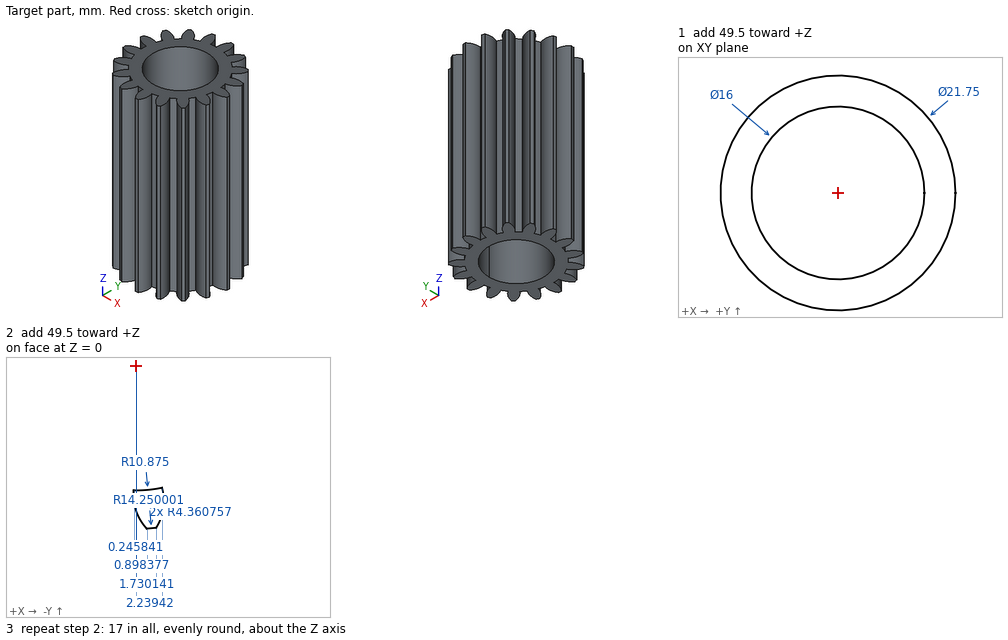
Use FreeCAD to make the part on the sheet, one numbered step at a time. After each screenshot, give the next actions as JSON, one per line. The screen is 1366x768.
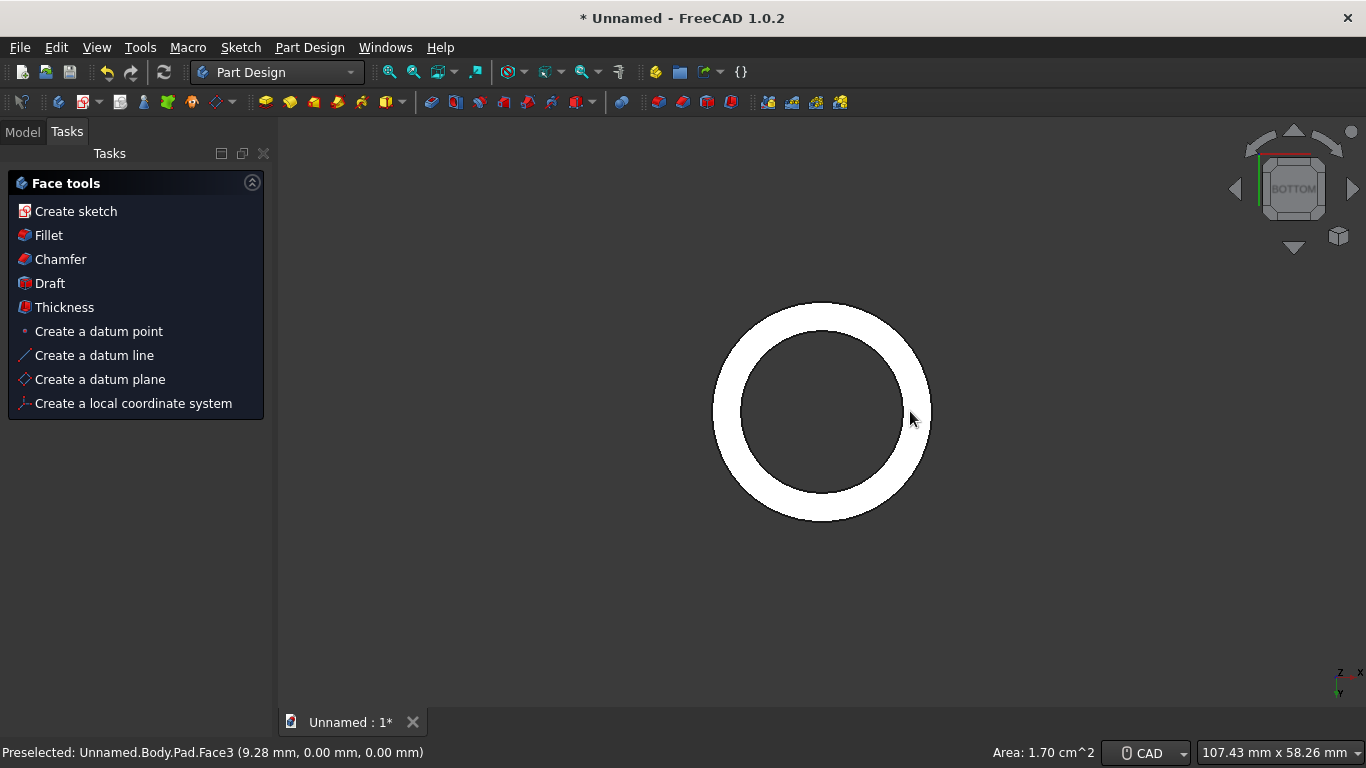
{"action": "left_click", "coordinate": [84, 102]}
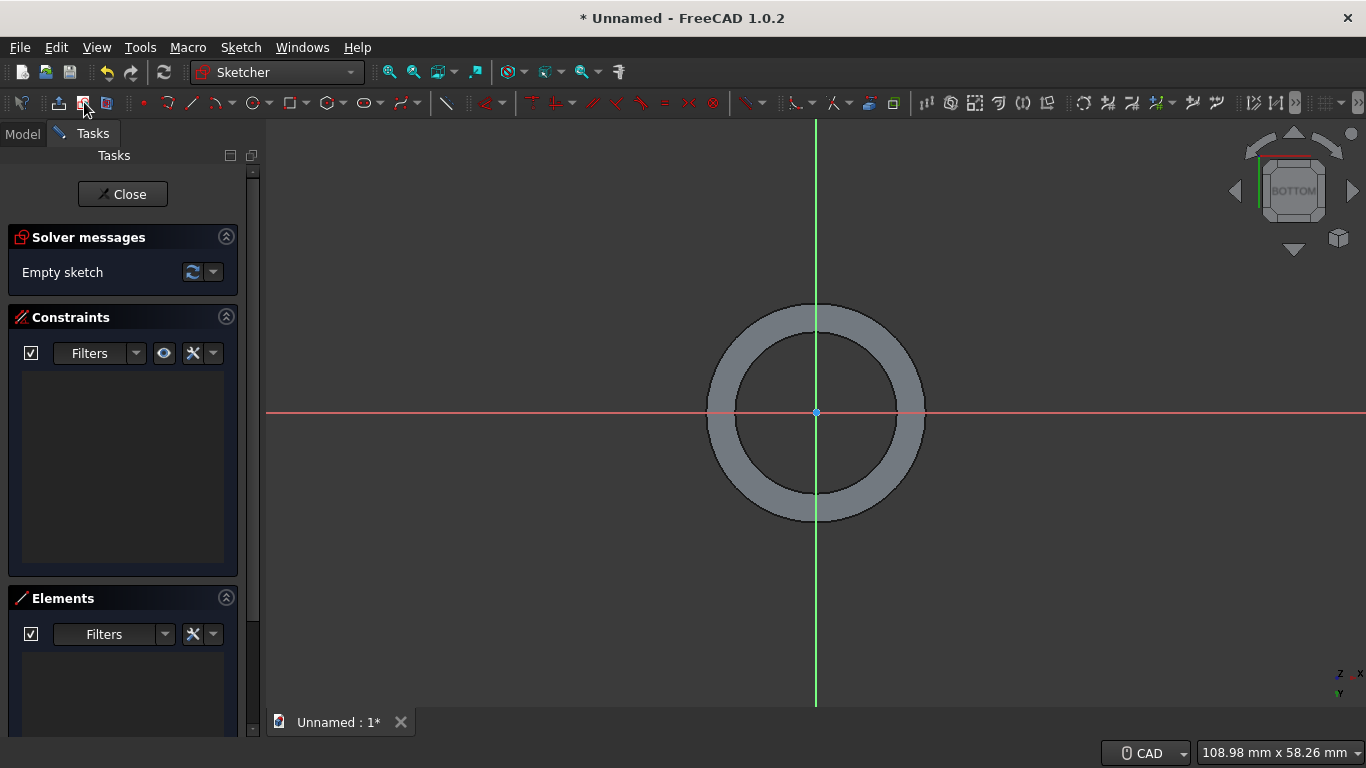
{"action": "scroll", "coordinate": [835, 551], "scroll_direction": "up", "scroll_amount": 12}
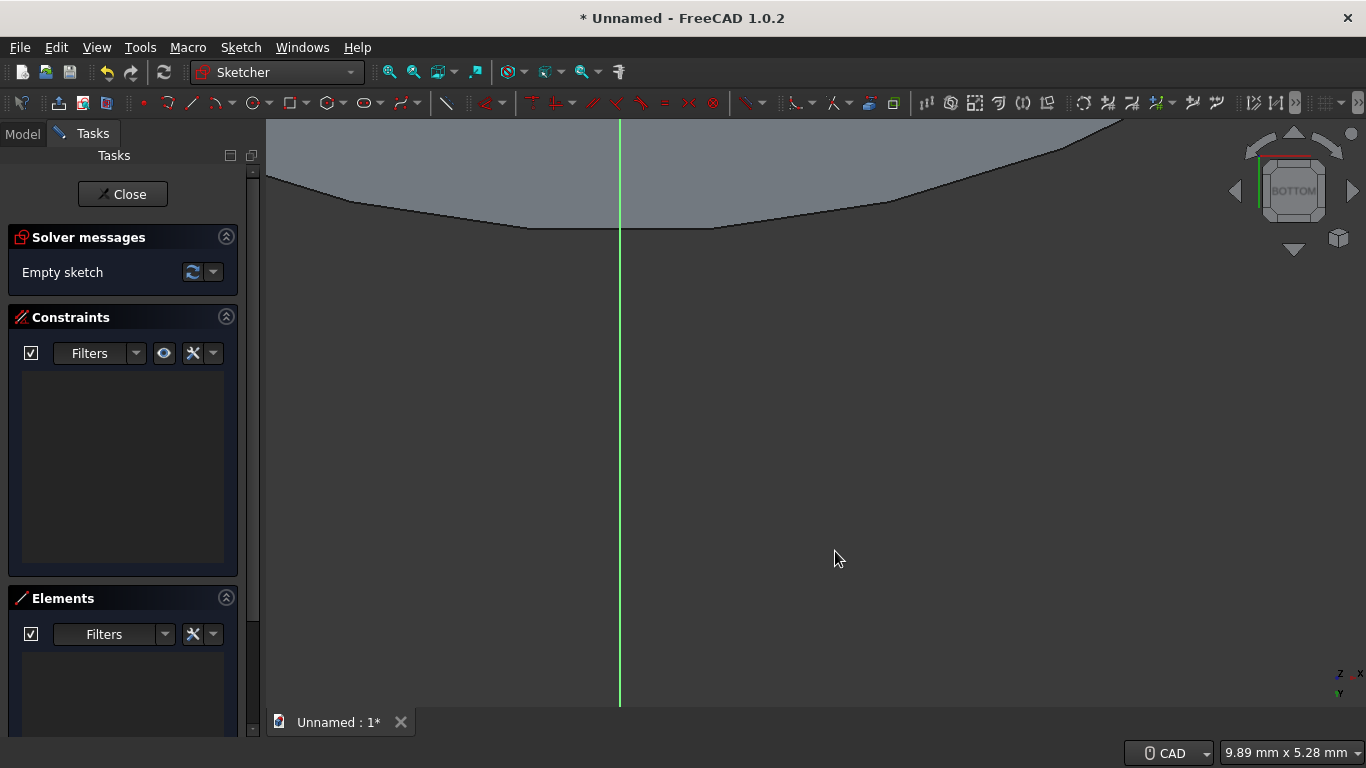
{"action": "key", "text": "g 3 a"}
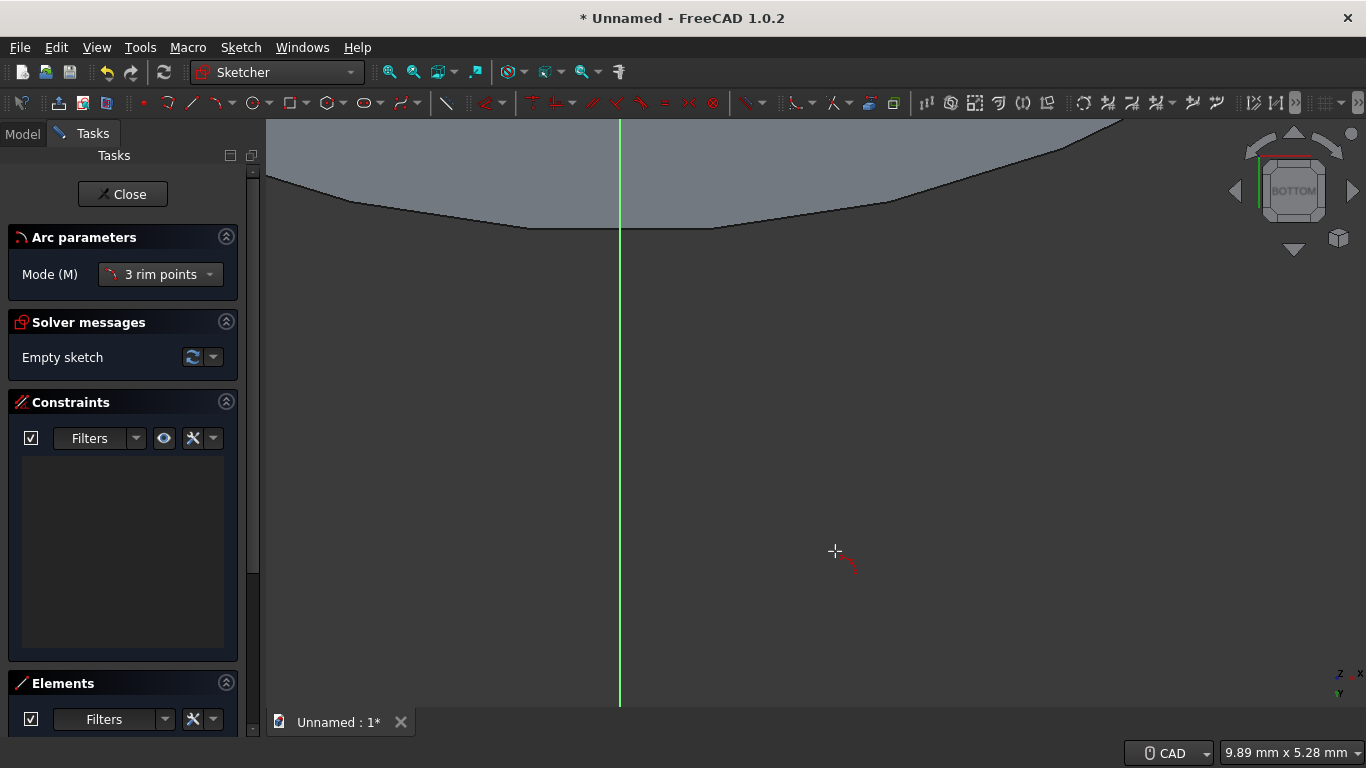
{"action": "left_click", "coordinate": [593, 232]}
{"action": "left_click", "coordinate": [870, 206]}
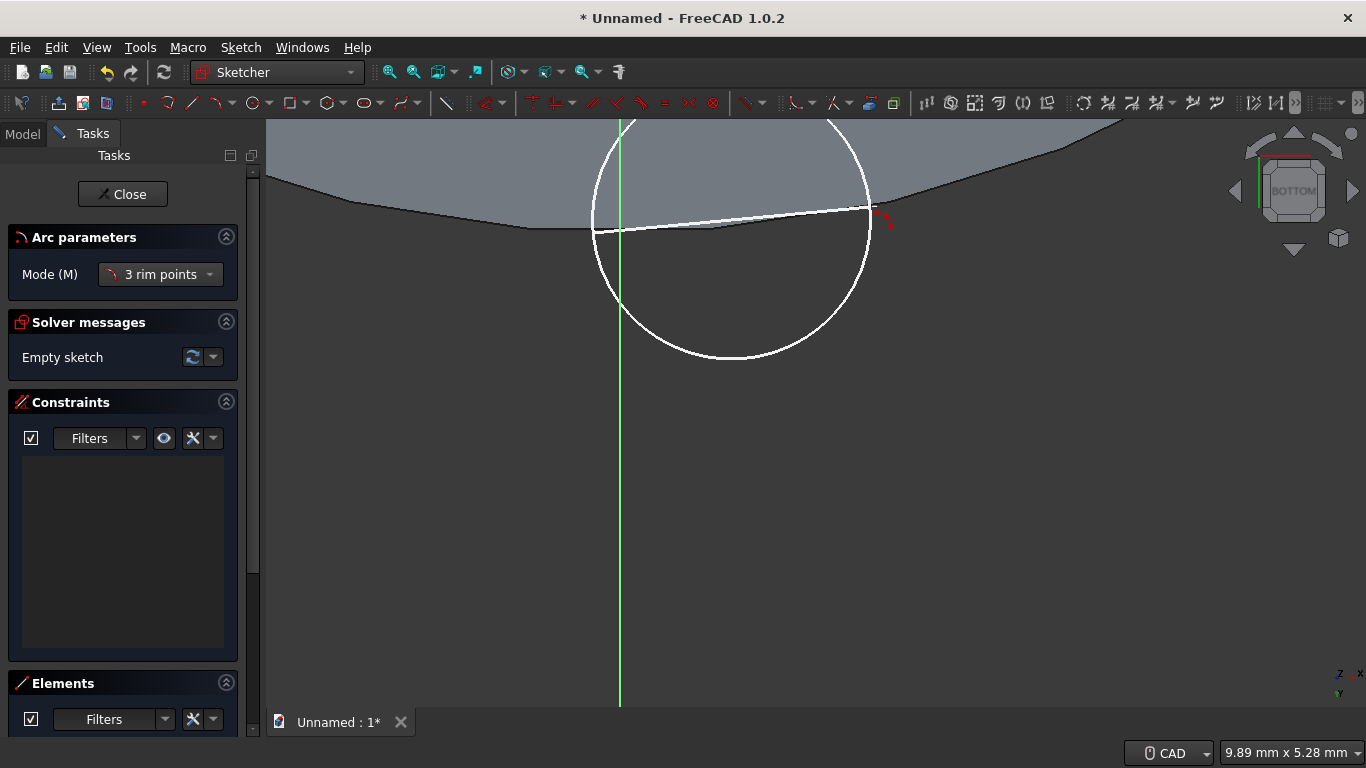
{"action": "scroll", "coordinate": [732, 227], "scroll_direction": "up", "scroll_amount": 4}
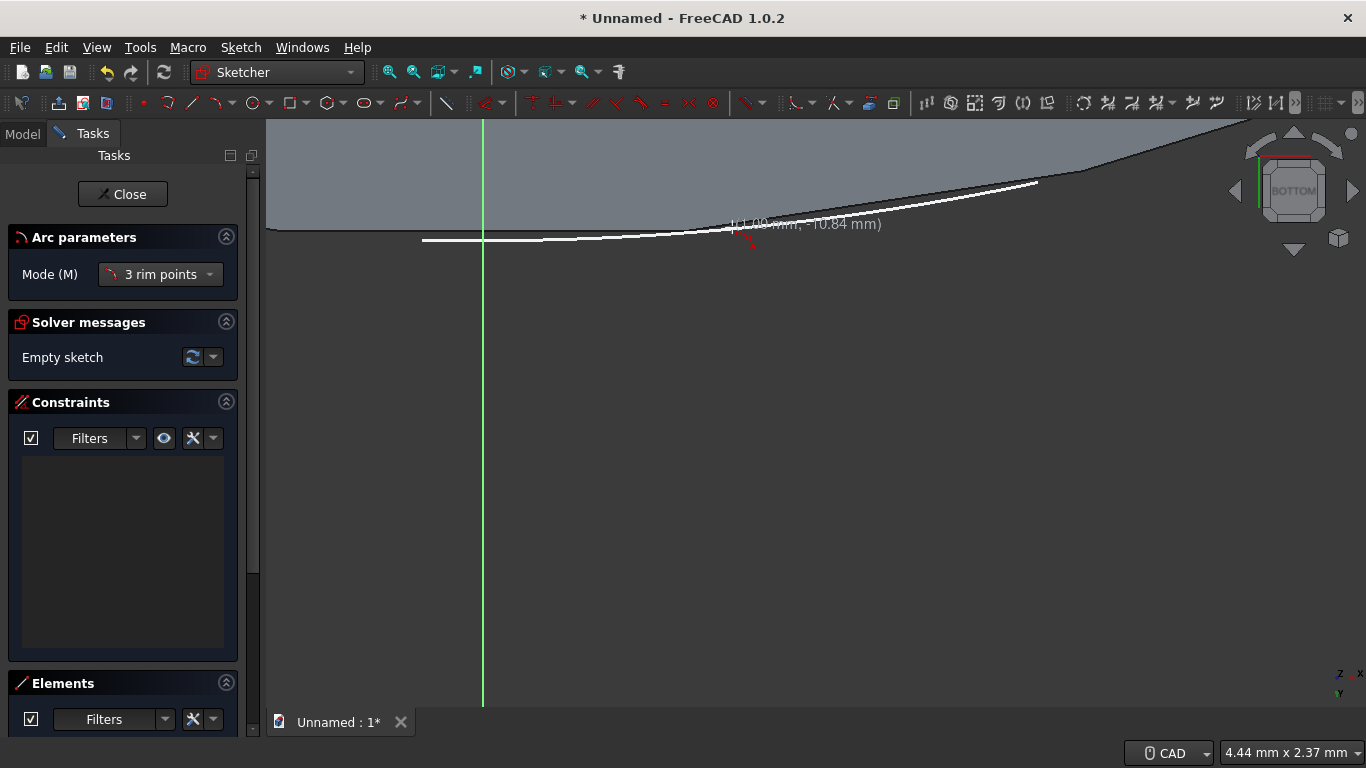
{"action": "left_click", "coordinate": [732, 227]}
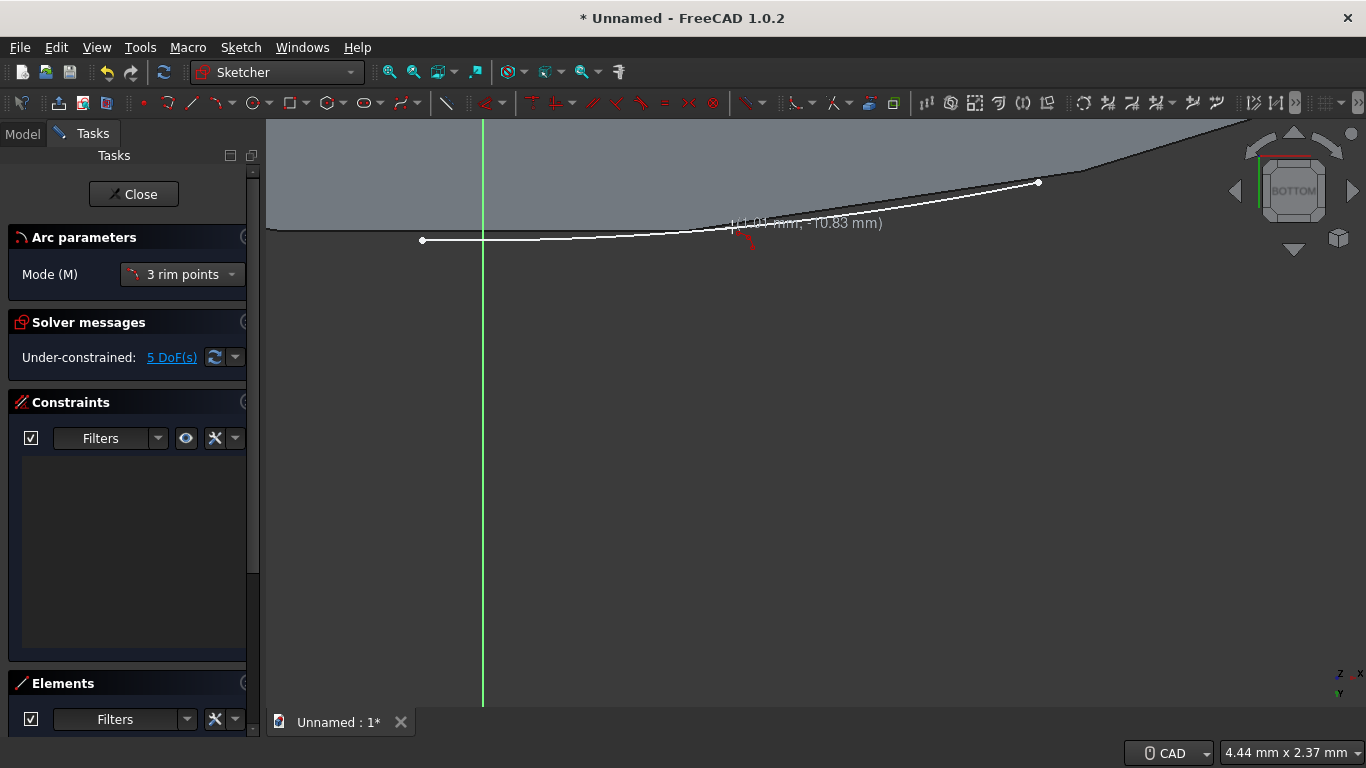
{"action": "left_click", "coordinate": [1039, 182]}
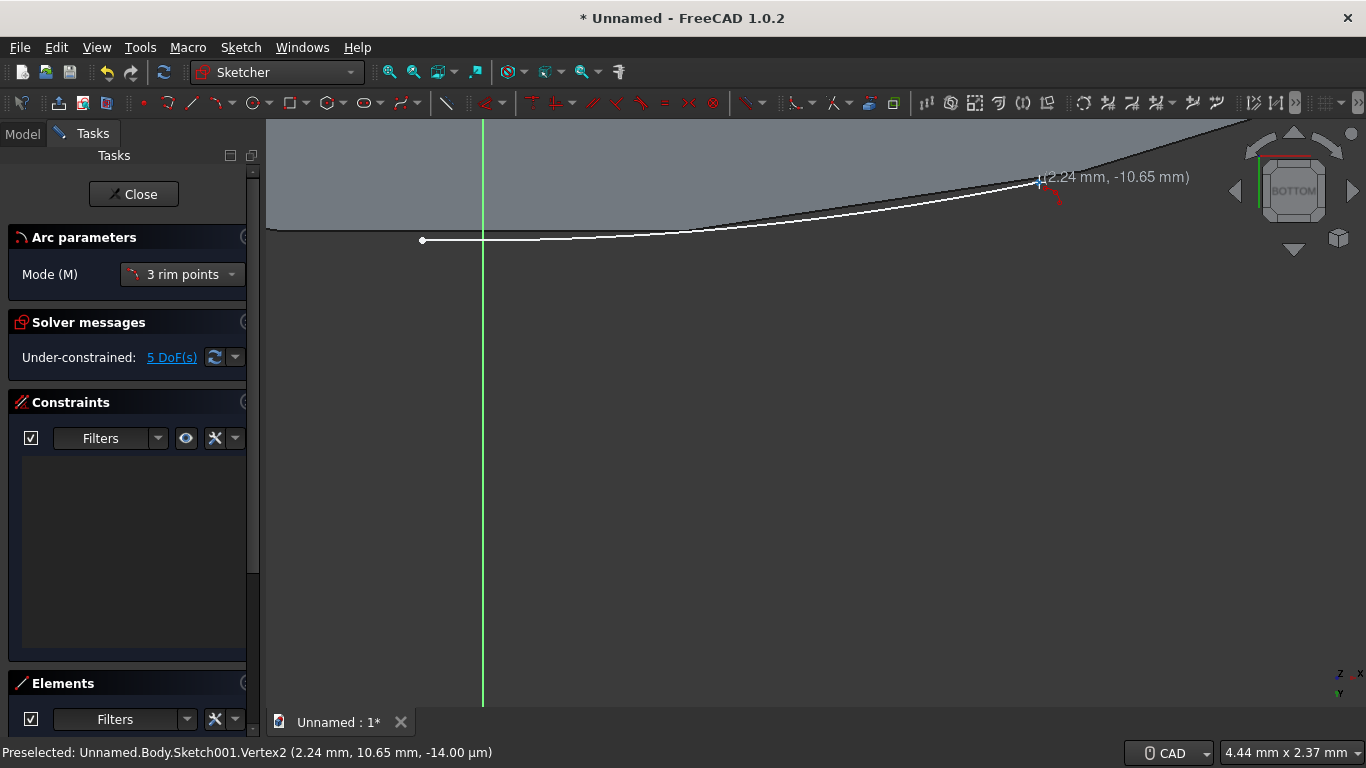
{"action": "scroll", "coordinate": [750, 241], "scroll_direction": "down", "scroll_amount": 4}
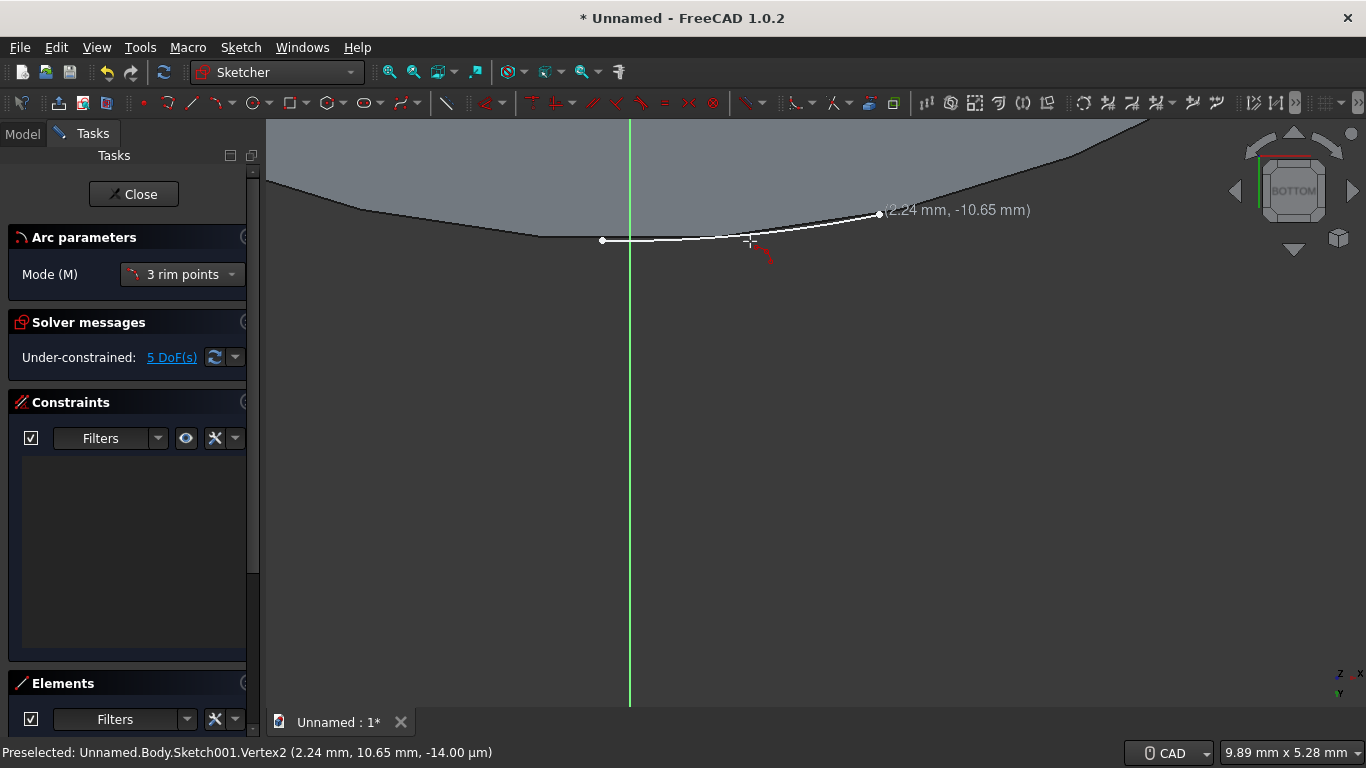
{"action": "left_click", "coordinate": [823, 604]}
{"action": "left_click", "coordinate": [892, 415]}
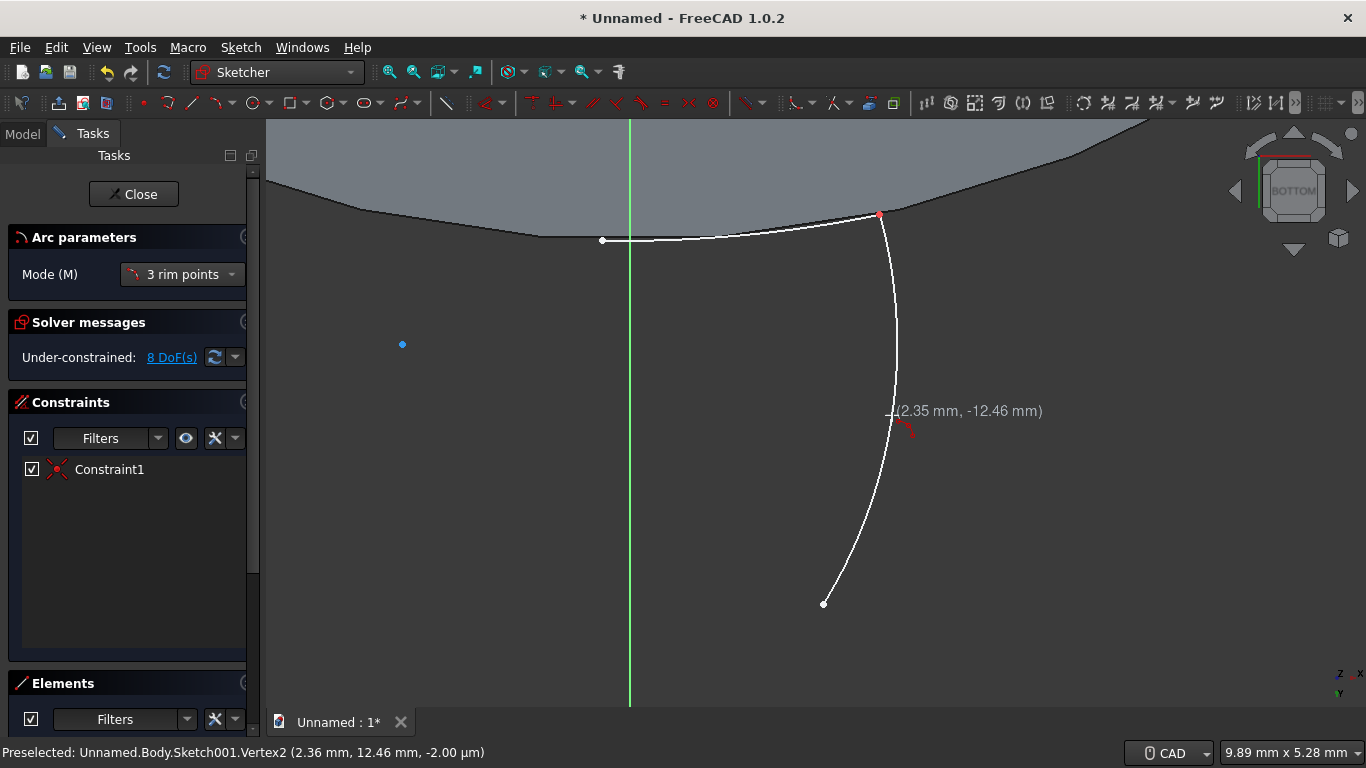
{"action": "left_click", "coordinate": [823, 605]}
{"action": "left_click", "coordinate": [730, 612]}